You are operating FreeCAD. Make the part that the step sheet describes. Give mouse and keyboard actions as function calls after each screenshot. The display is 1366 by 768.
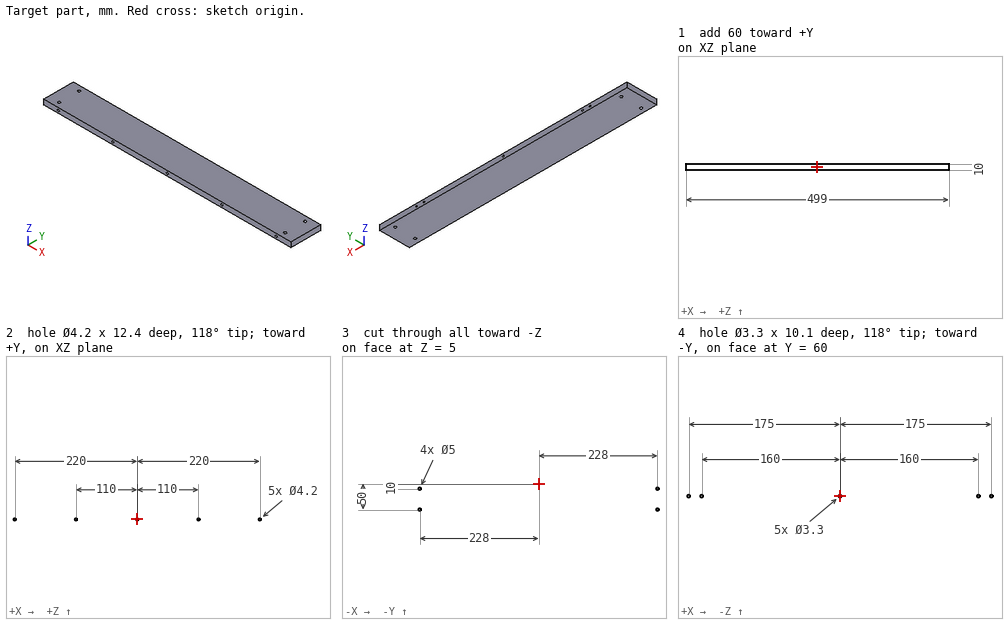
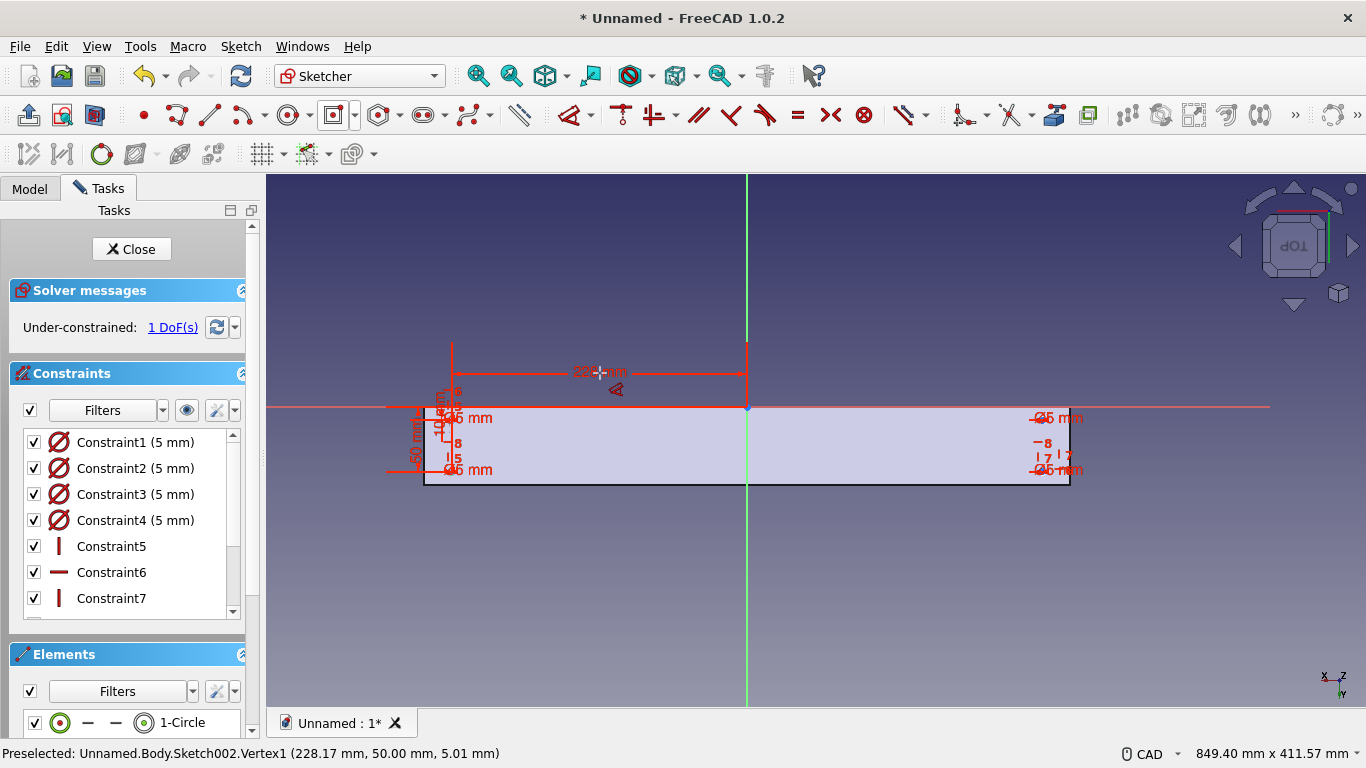
click(1043, 420)
click(895, 373)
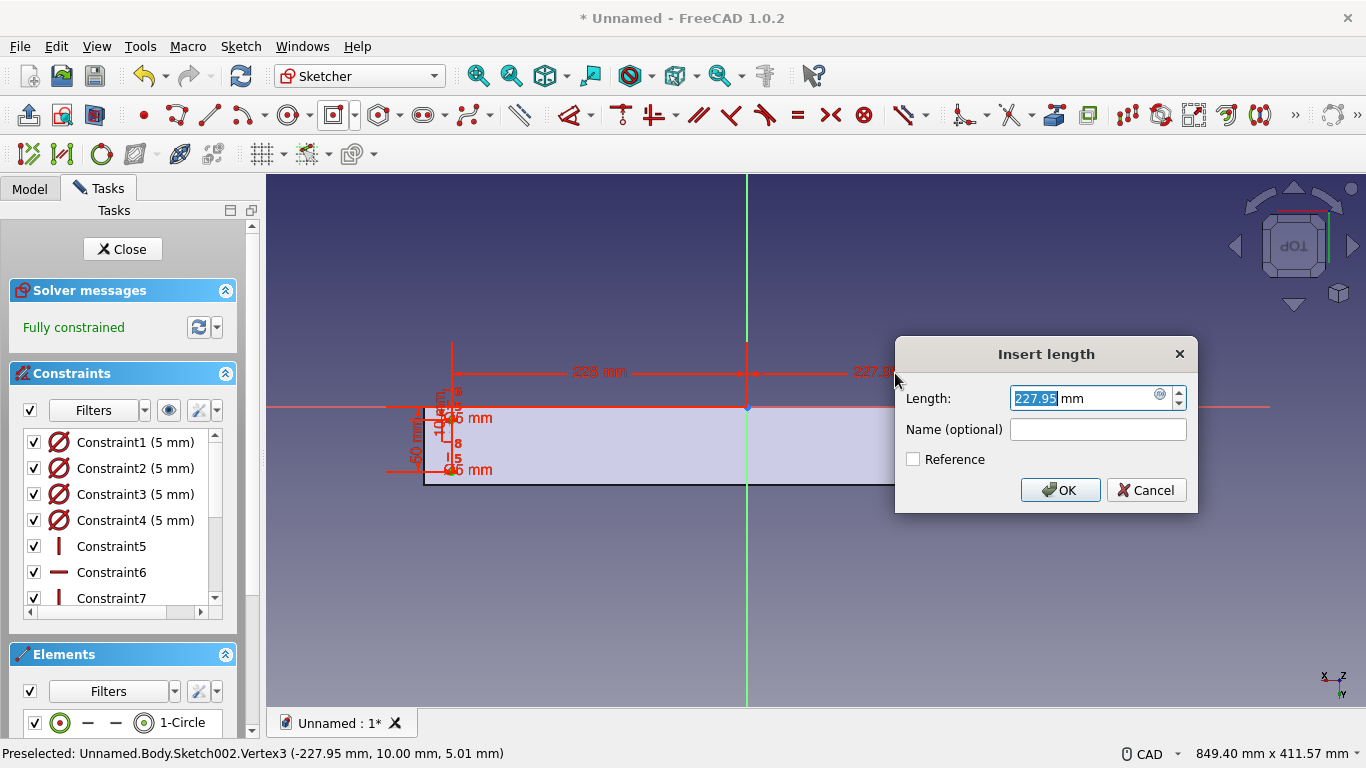
text(228)
key(Return)
key(Escape)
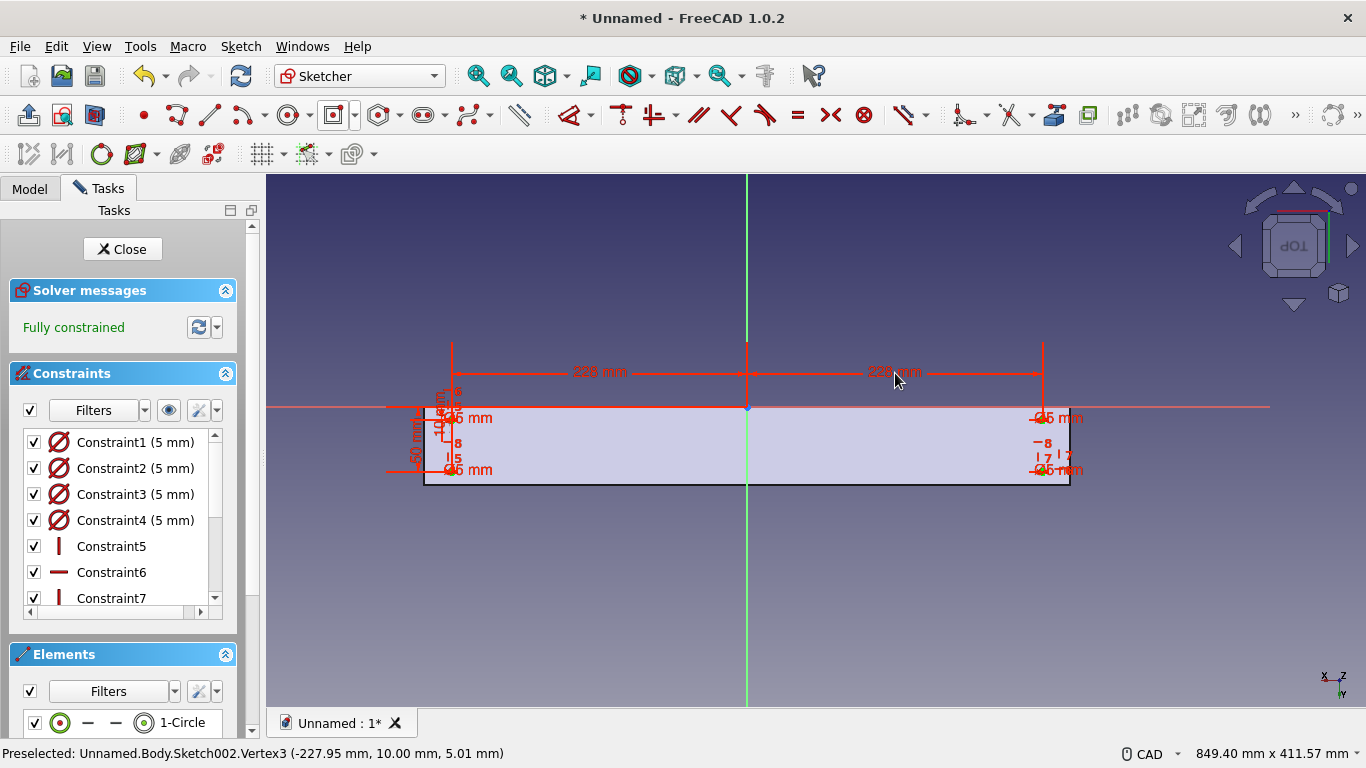
click(123, 249)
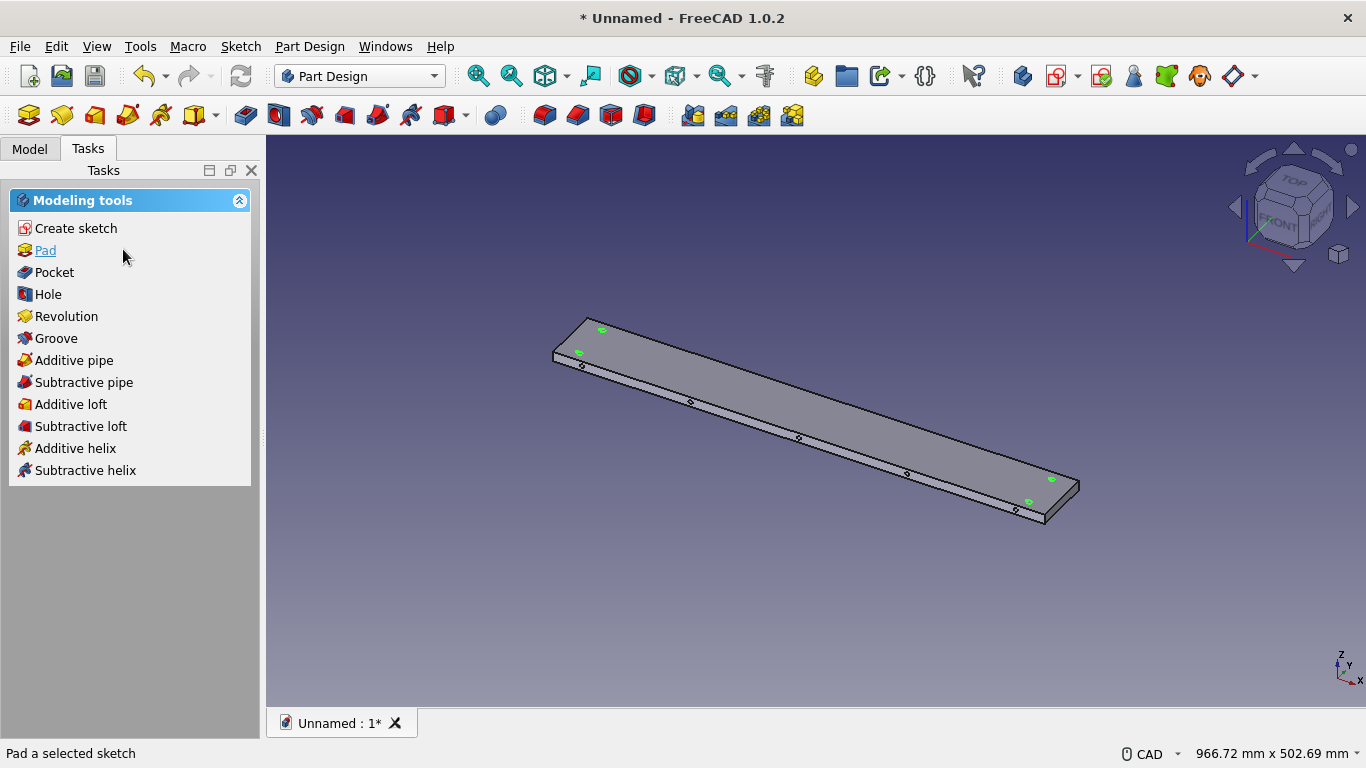
click(246, 116)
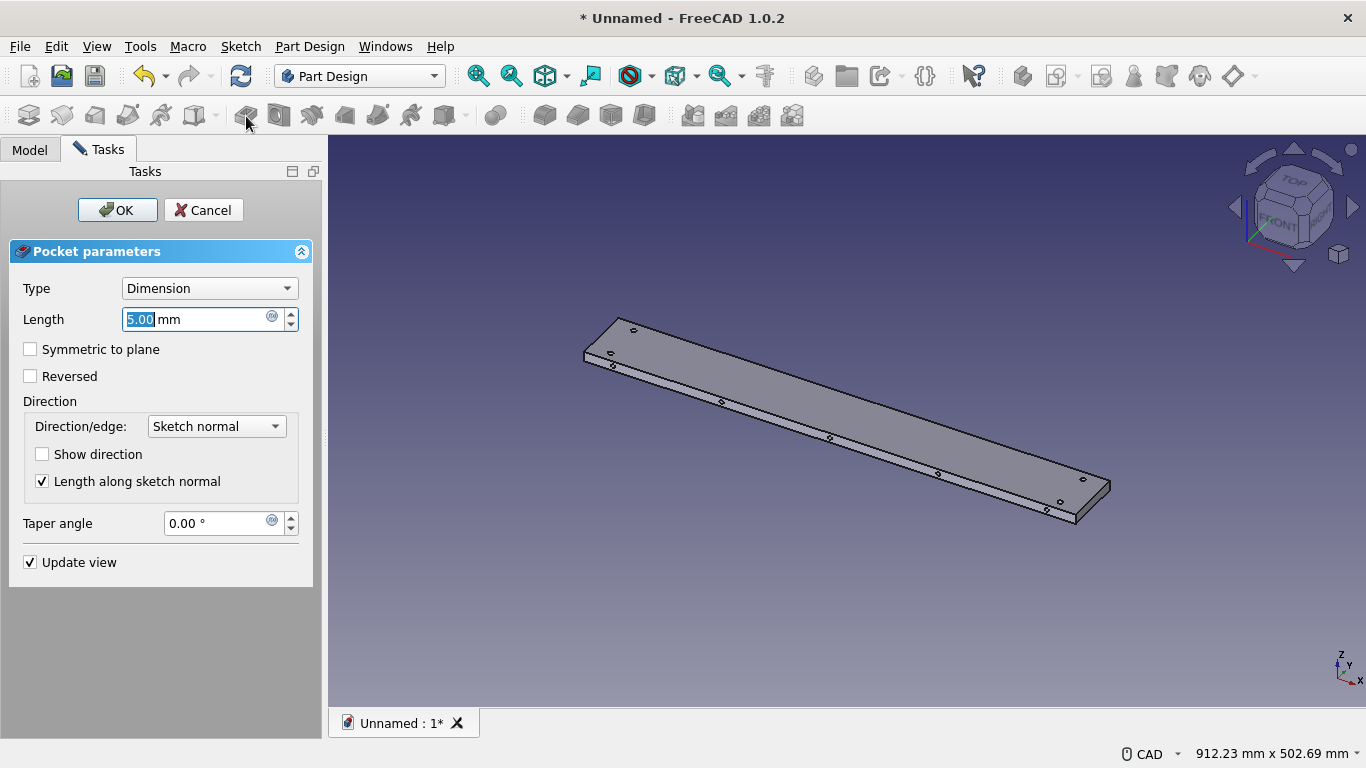
click(210, 288)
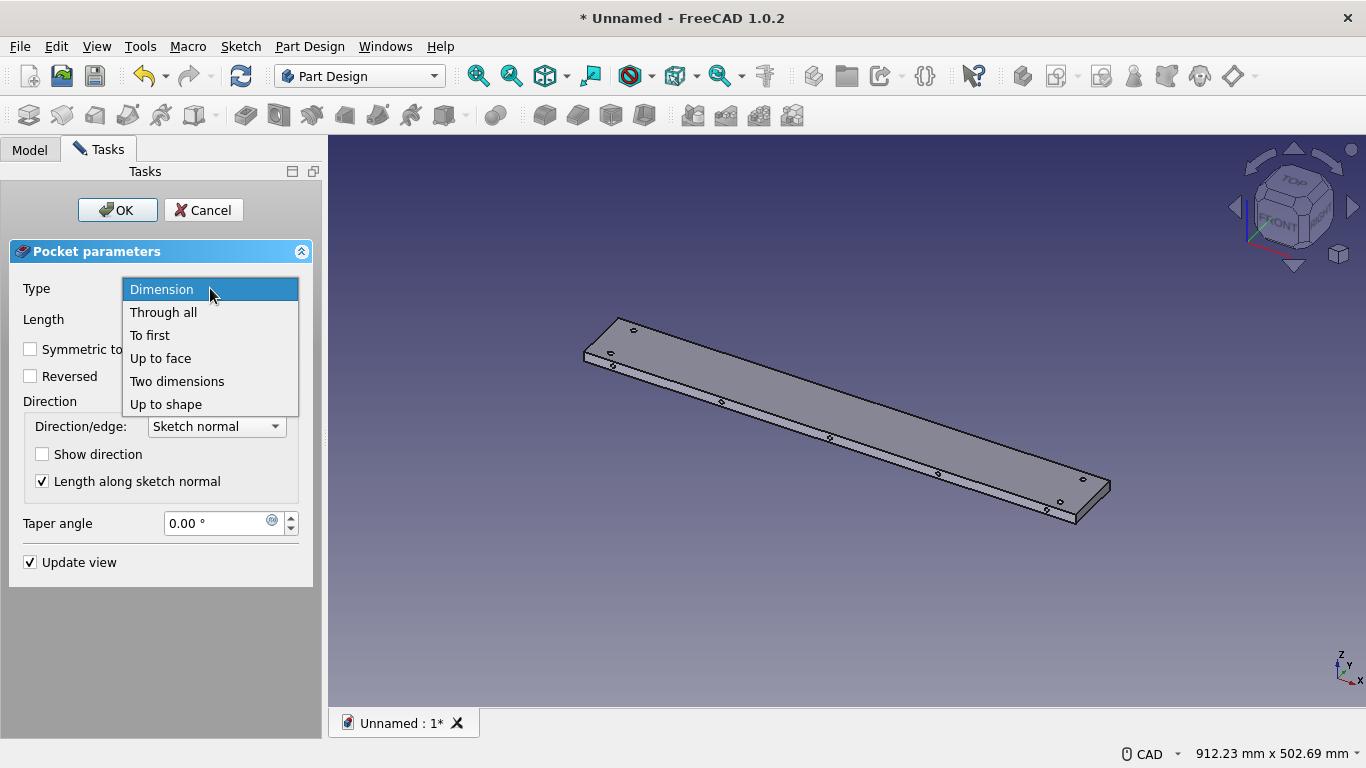
click(208, 312)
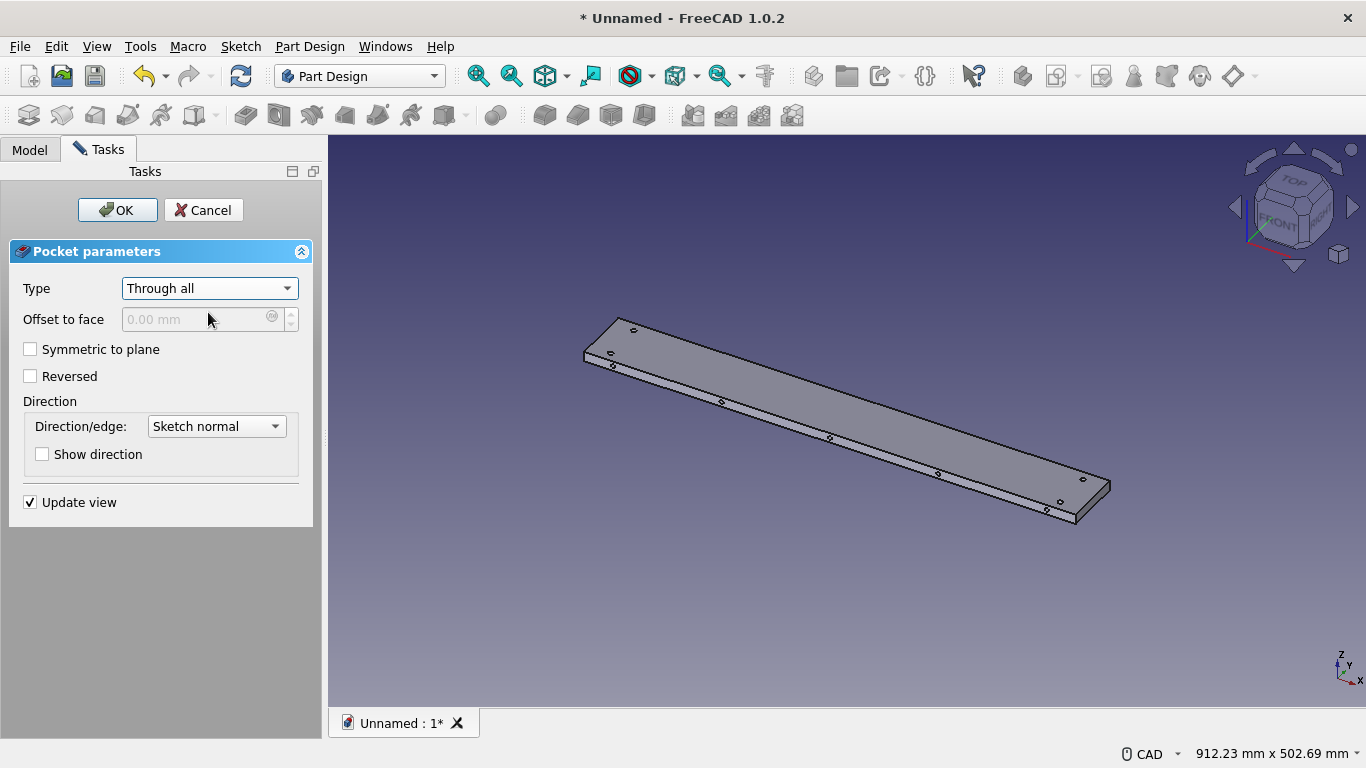
click(118, 210)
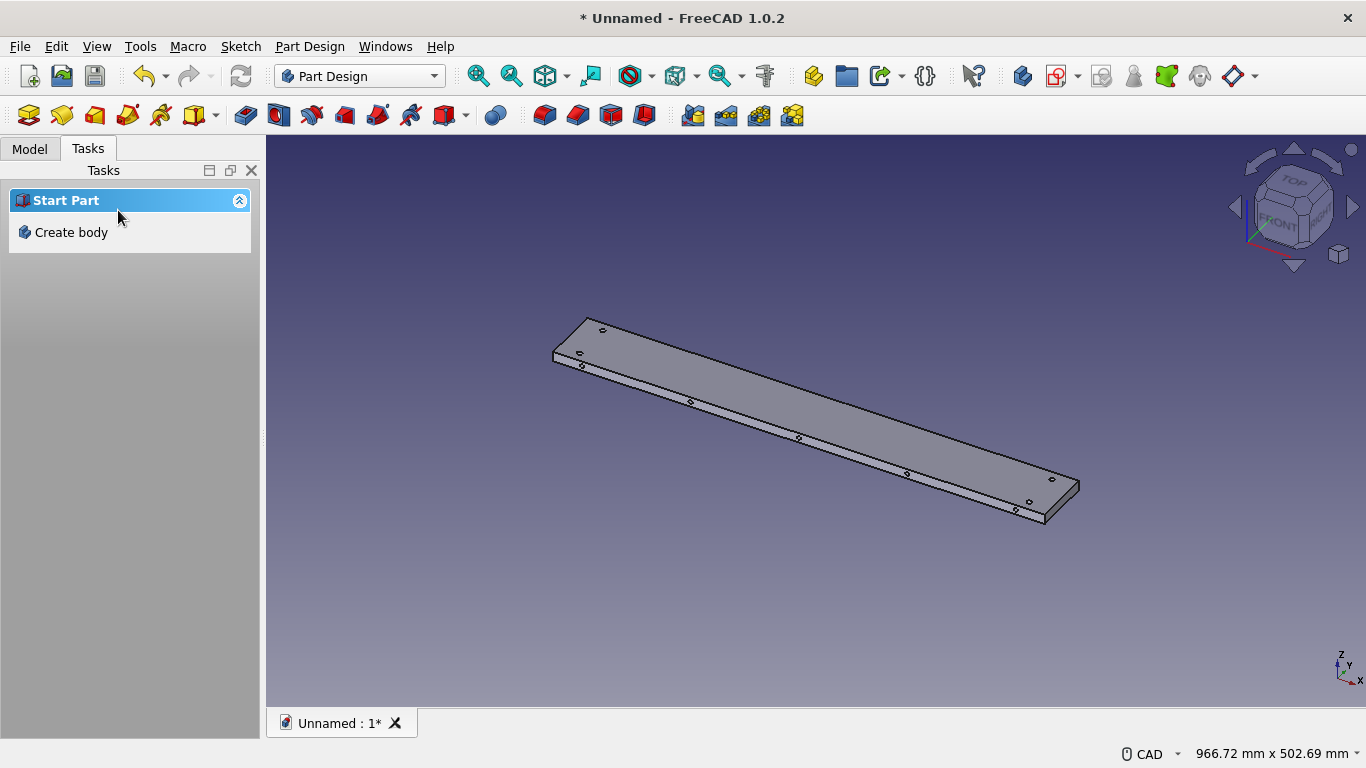
key(4)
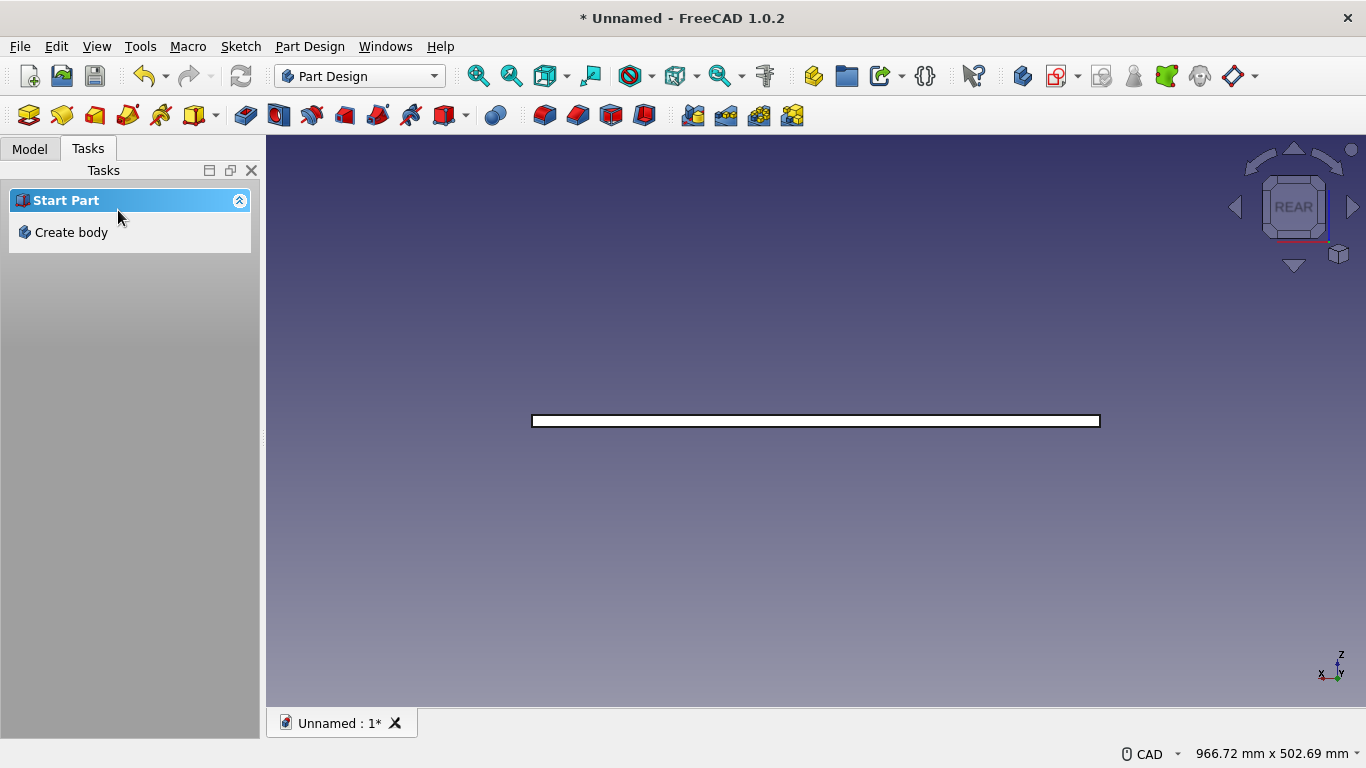
scroll(573, 420, up, 4)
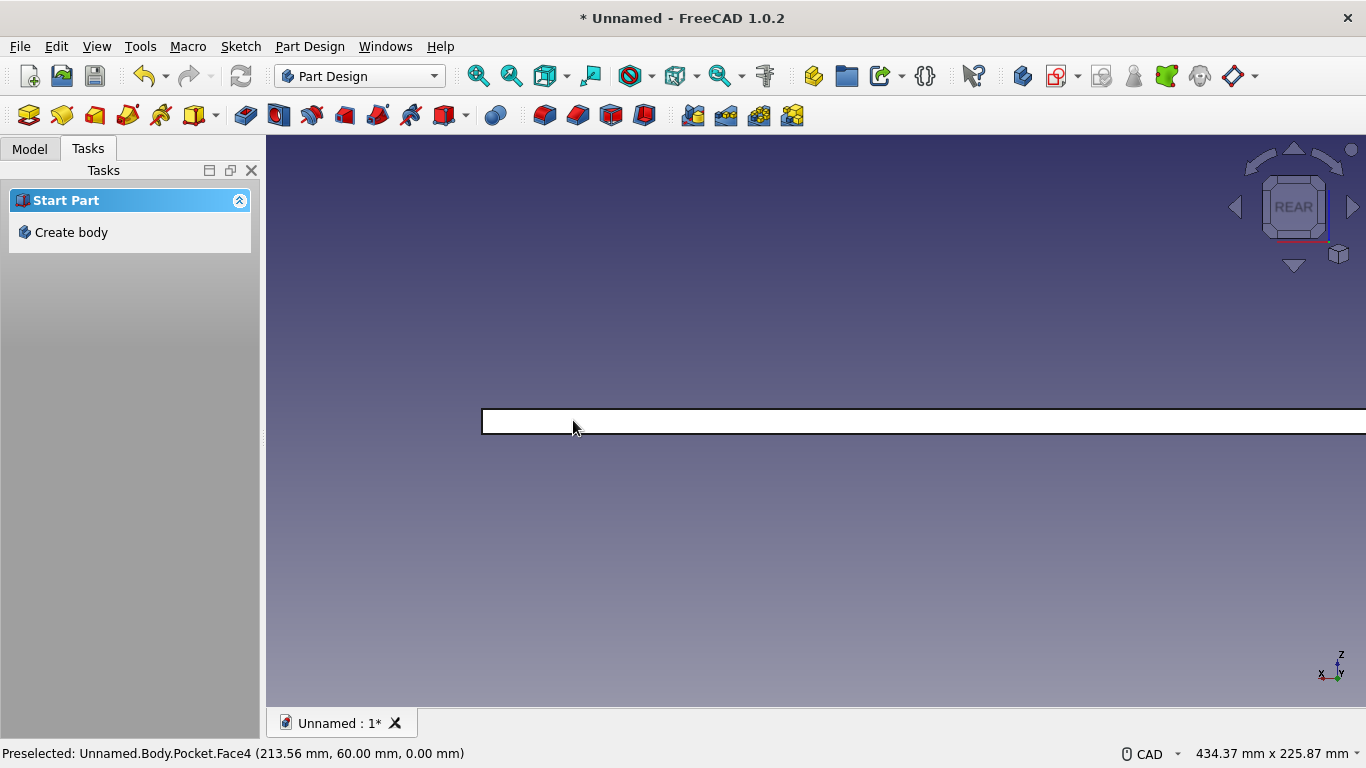
click(572, 421)